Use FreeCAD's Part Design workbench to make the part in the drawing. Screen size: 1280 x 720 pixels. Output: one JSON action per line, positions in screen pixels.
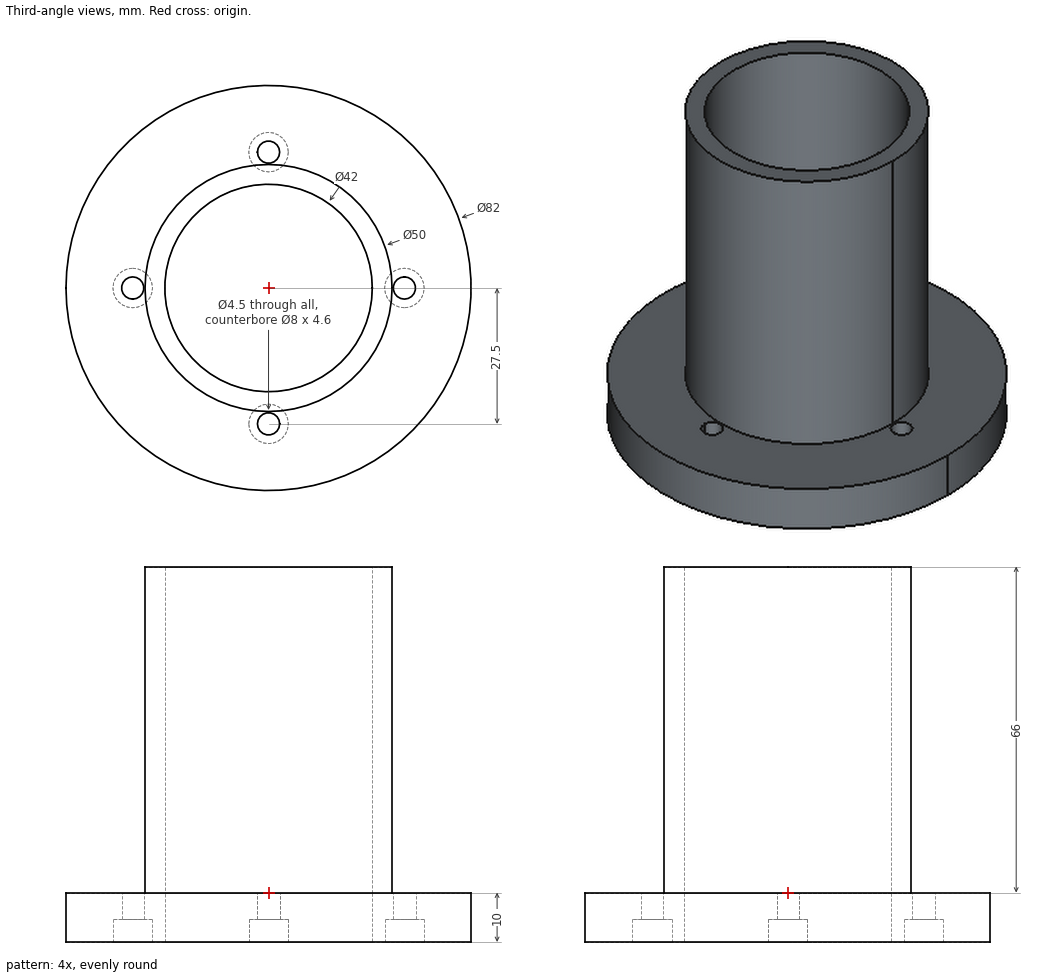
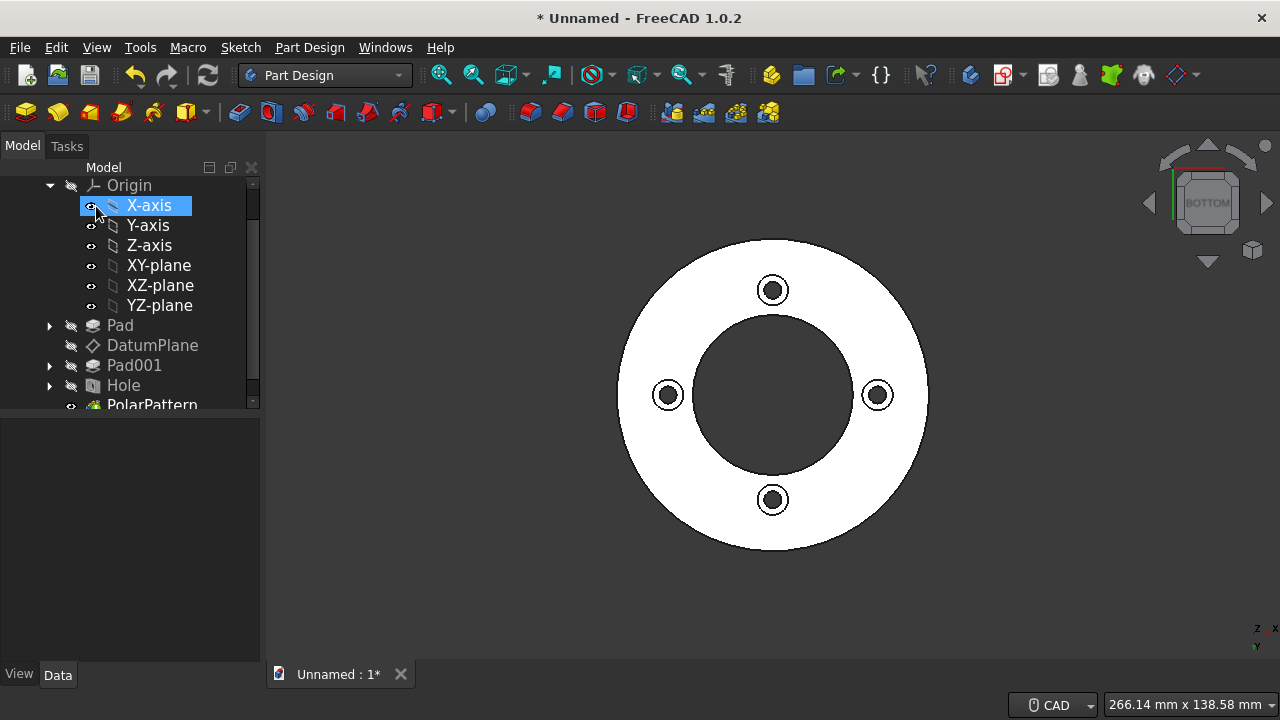
{"action": "key", "text": "0"}